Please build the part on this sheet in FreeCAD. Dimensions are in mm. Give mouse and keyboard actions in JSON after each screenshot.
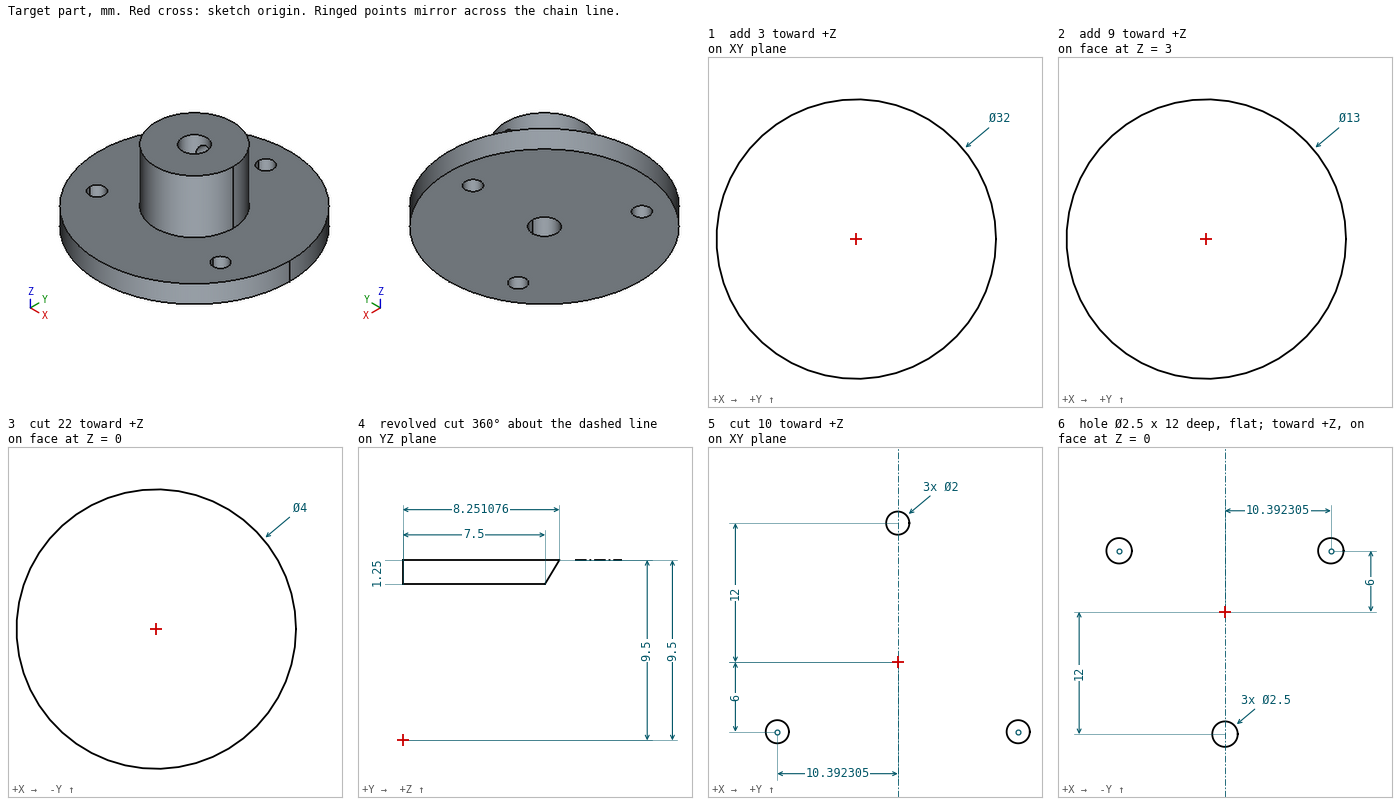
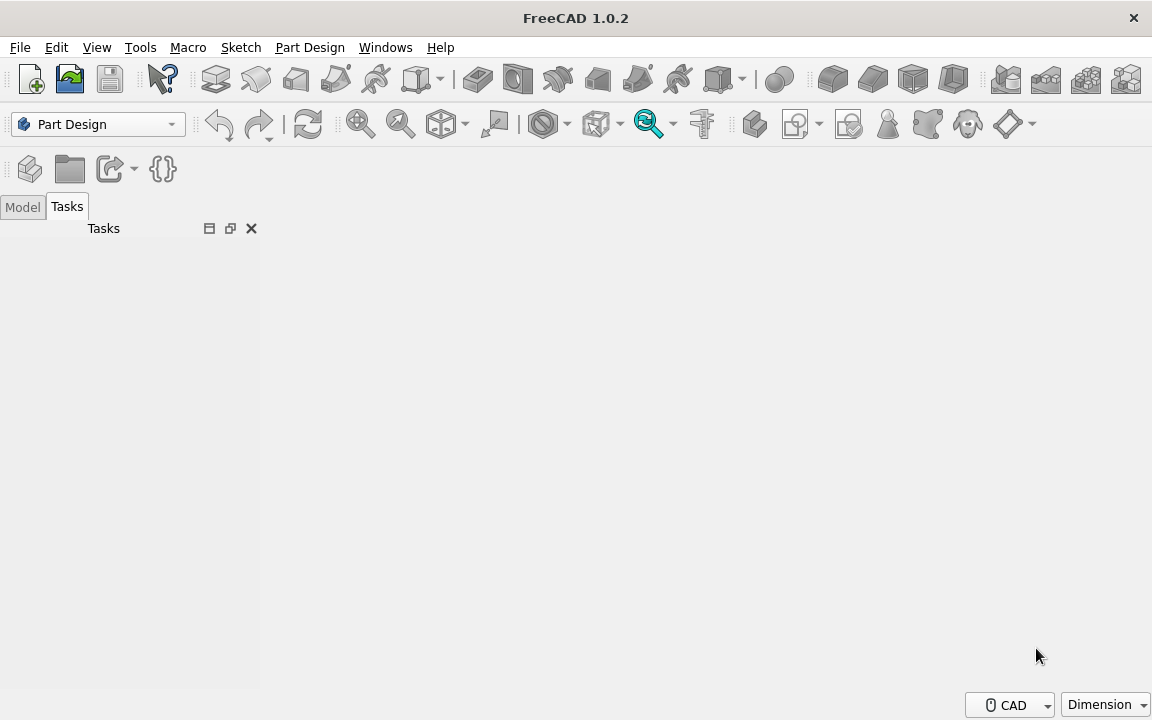
{"action": "left_click", "coordinate": [30, 80]}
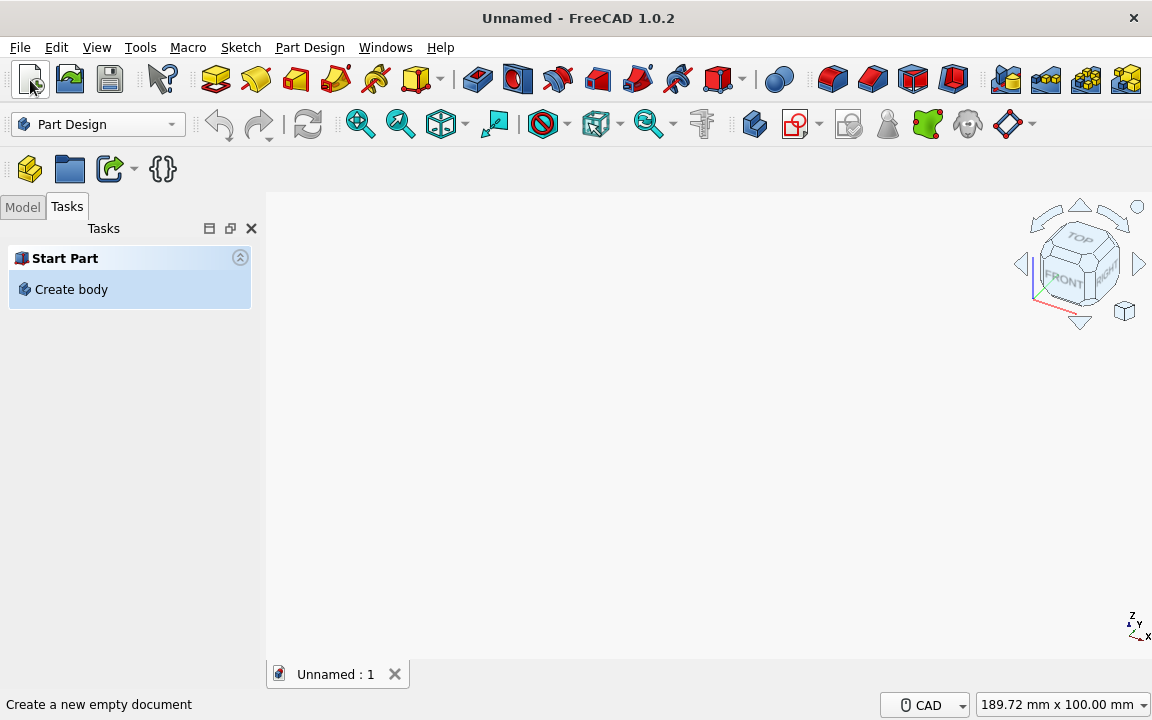
{"action": "left_click", "coordinate": [796, 124]}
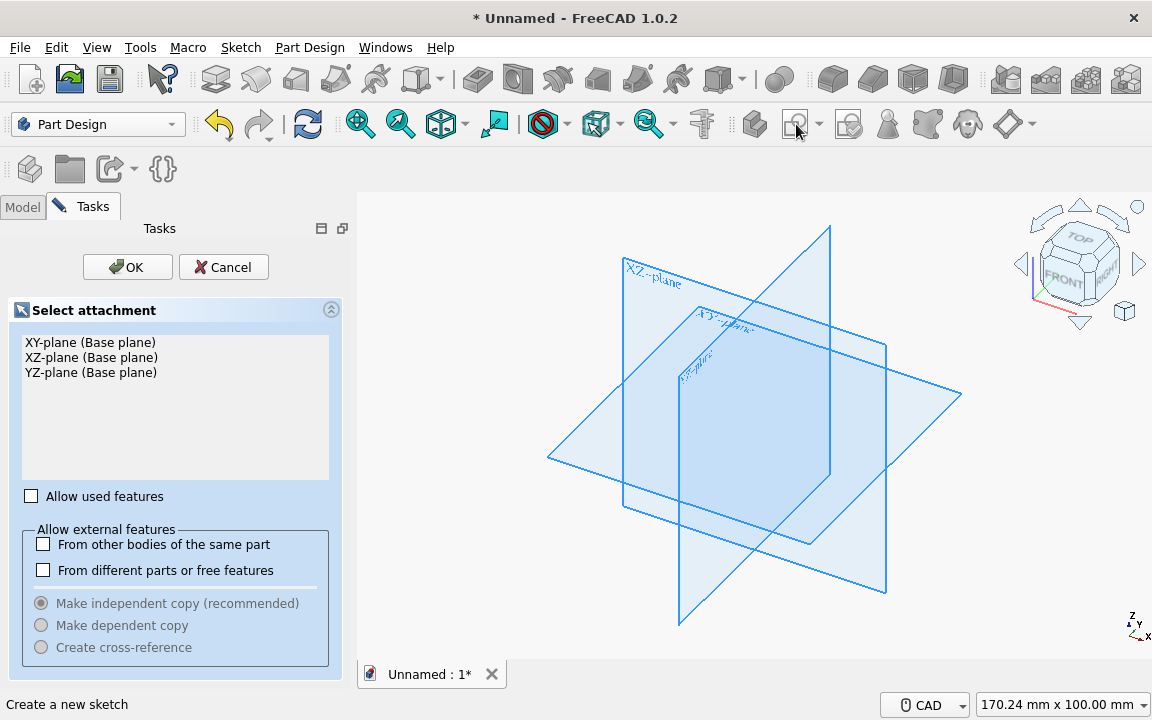
{"action": "left_click", "coordinate": [82, 342]}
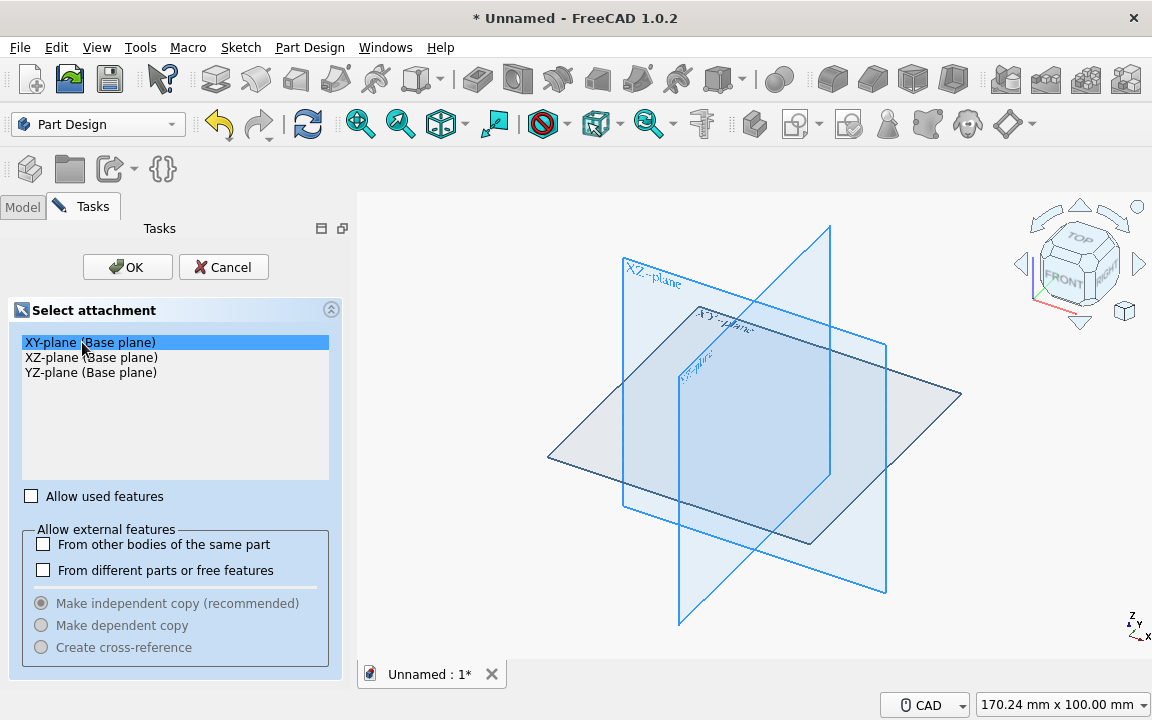
{"action": "left_click", "coordinate": [128, 267]}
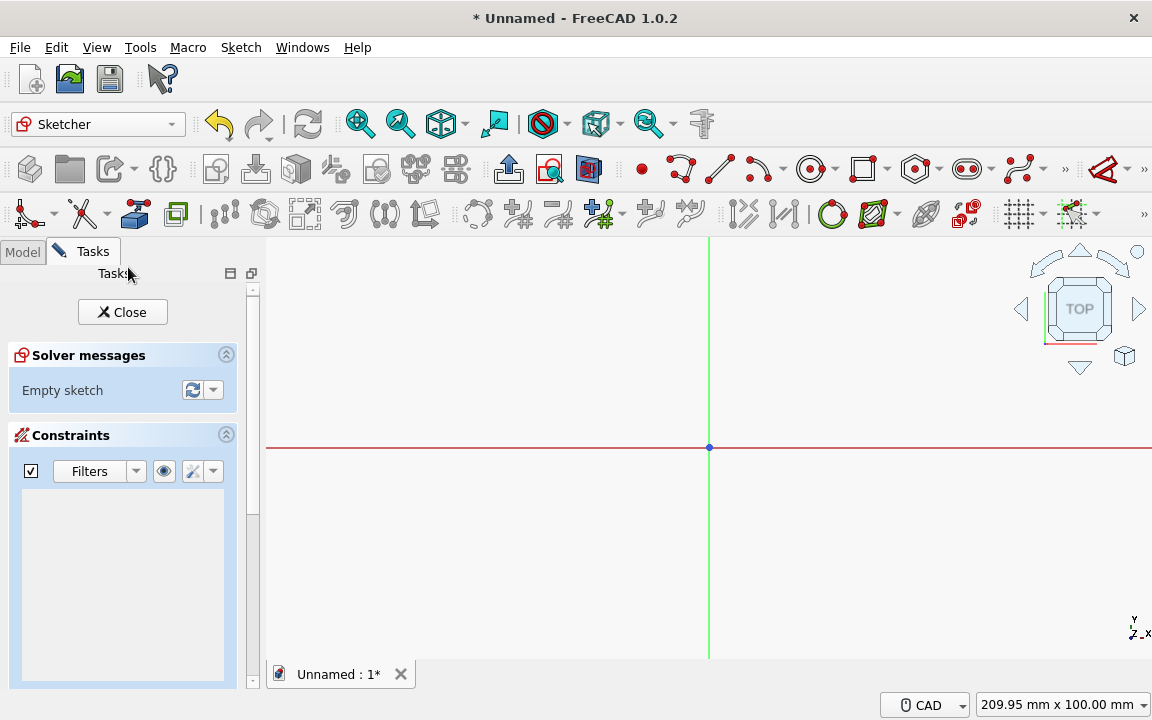
{"action": "scroll", "coordinate": [792, 448], "scroll_direction": "up", "scroll_amount": 3}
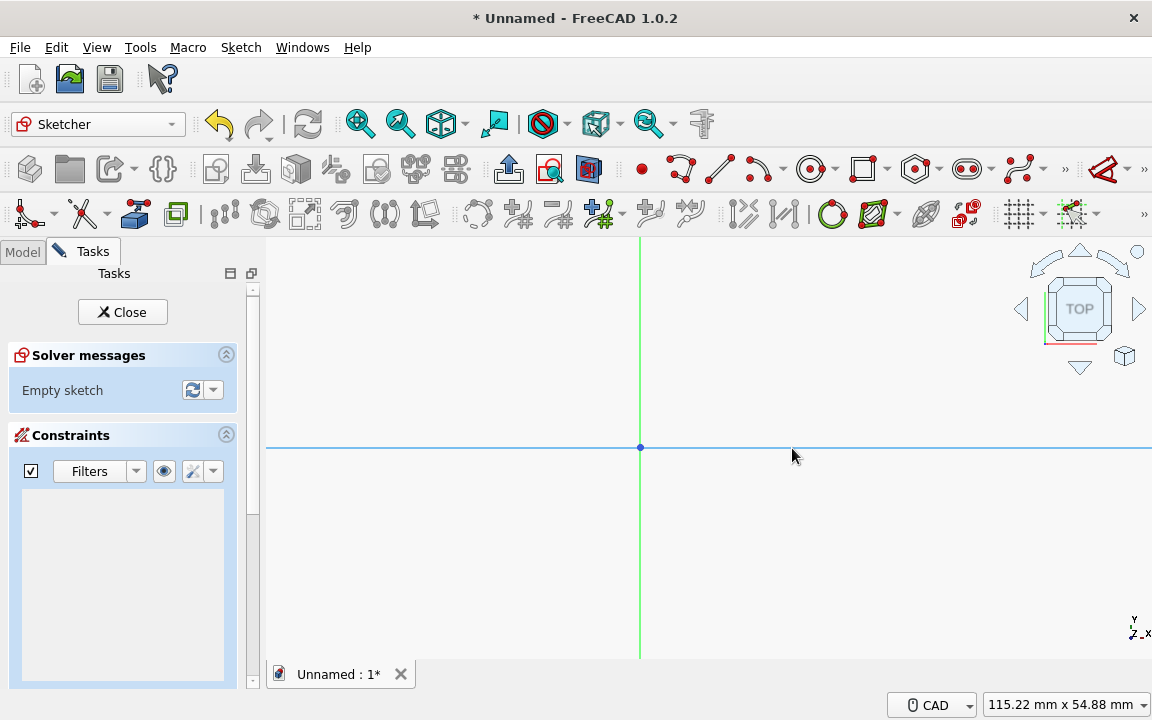
{"action": "left_click", "coordinate": [812, 170]}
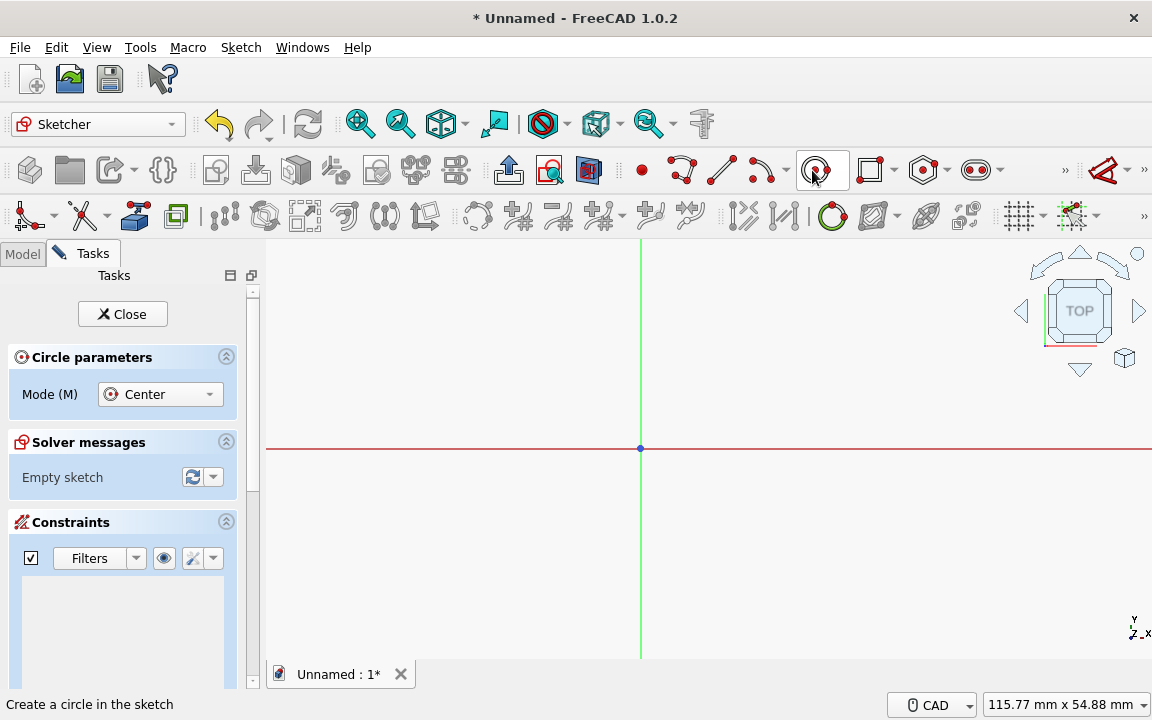
{"action": "left_click", "coordinate": [641, 449]}
{"action": "mouse_move", "coordinate": [727, 362]}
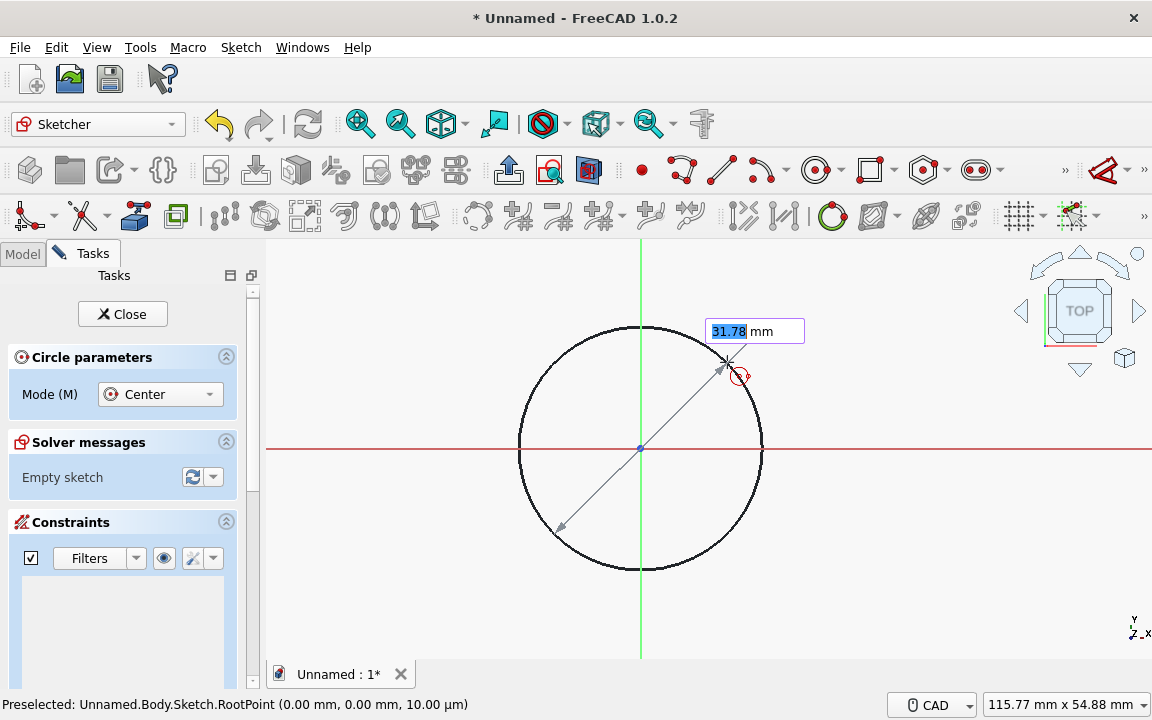
{"action": "type", "text": "32"}
{"action": "key", "text": "Return"}
{"action": "key", "text": "Escape"}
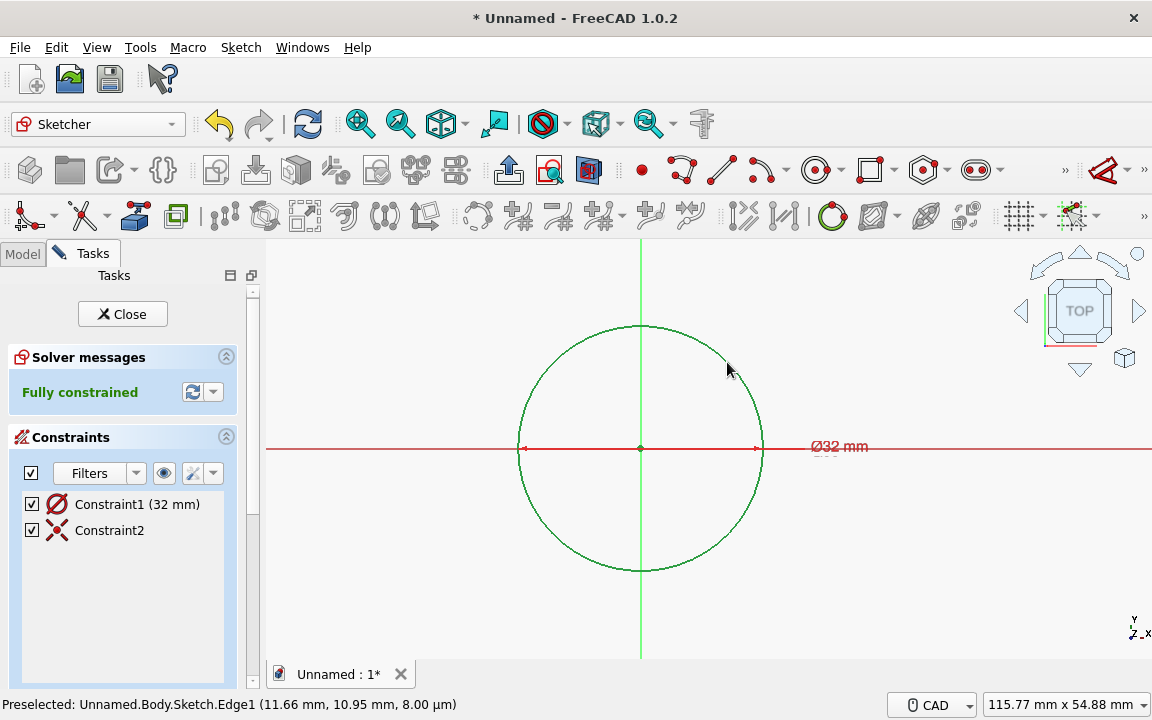
{"action": "left_click", "coordinate": [123, 314]}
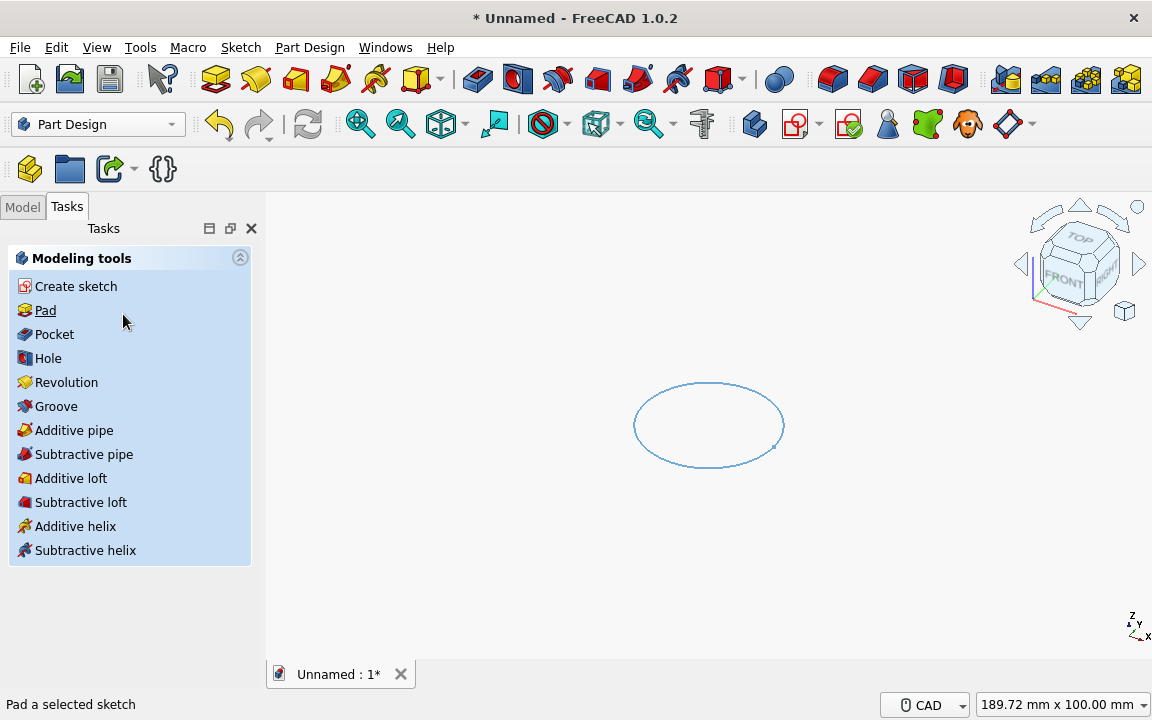
{"action": "left_click", "coordinate": [216, 80]}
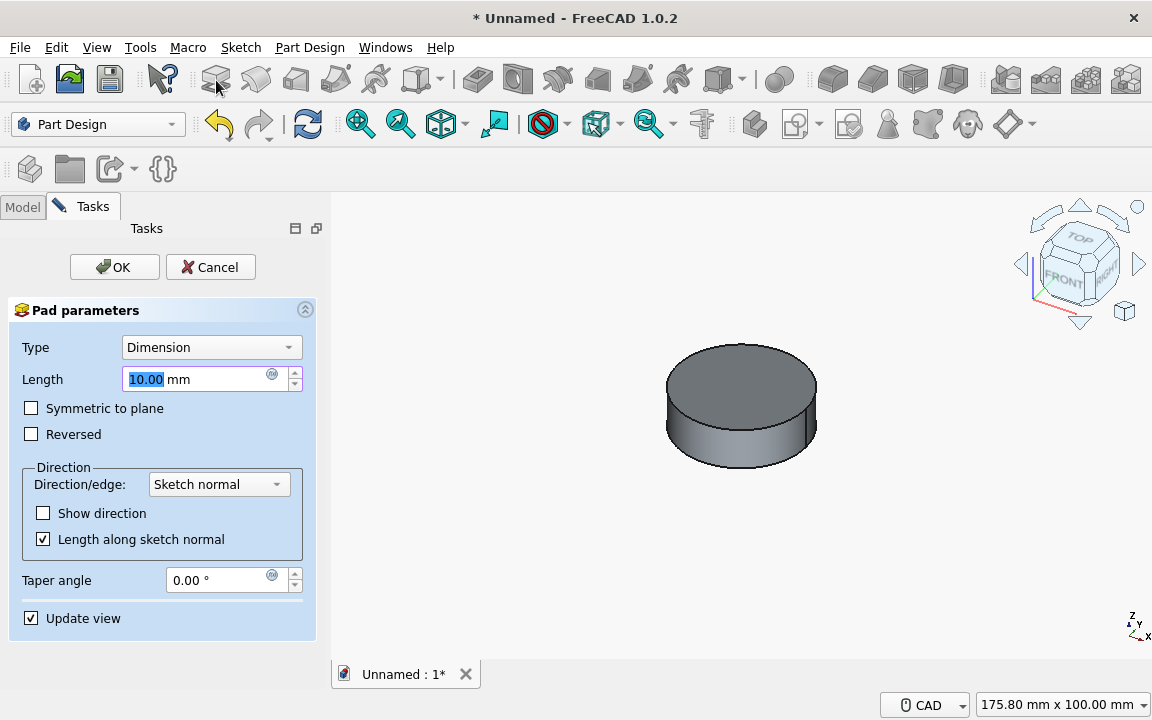
{"action": "type", "text": "3"}
{"action": "key", "text": "Tab"}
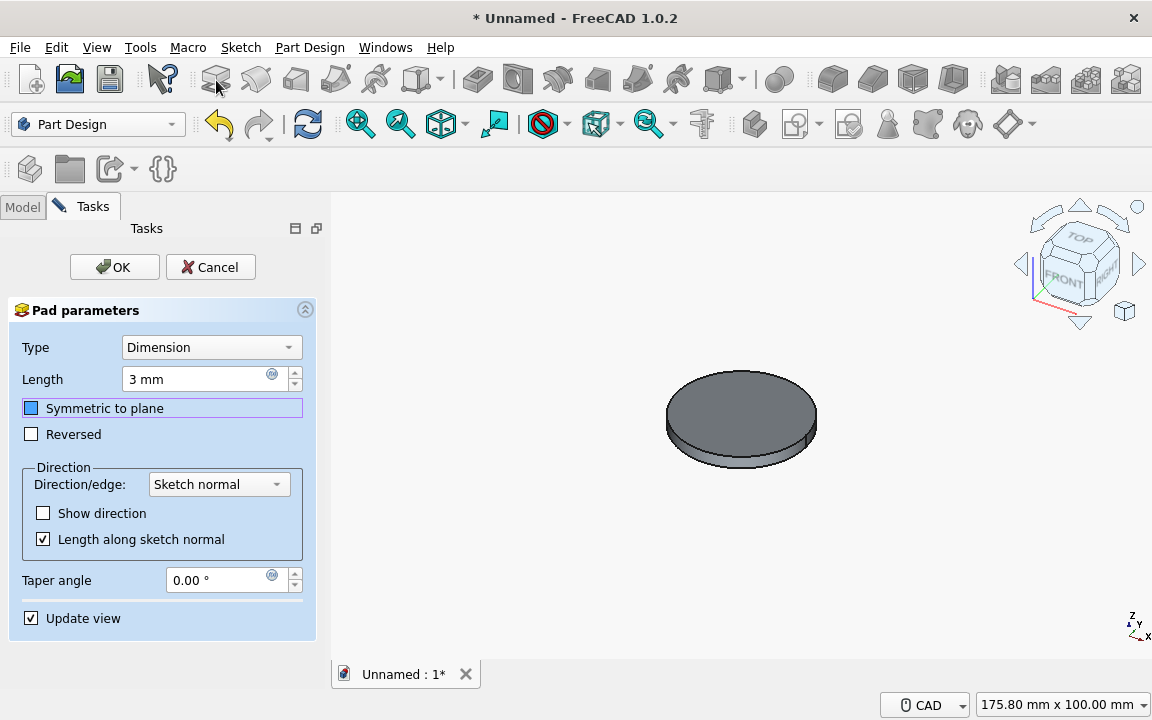
{"action": "left_click", "coordinate": [115, 267]}